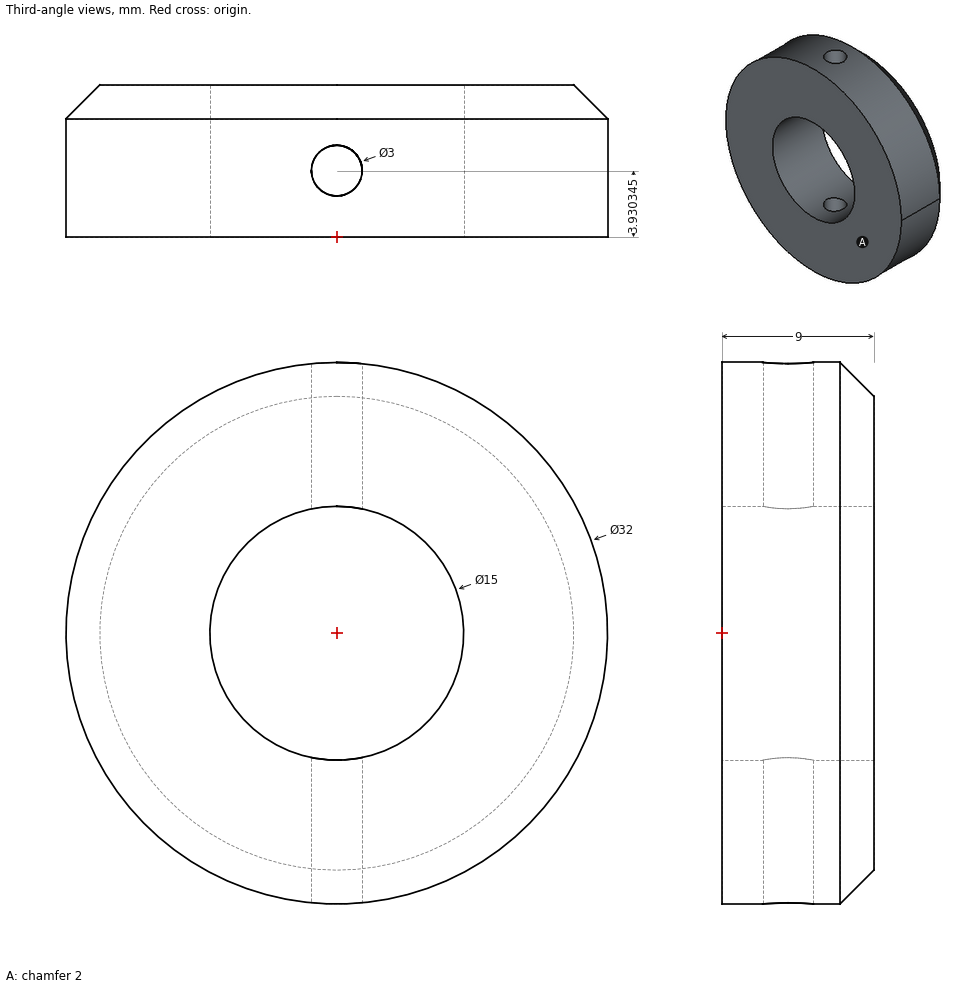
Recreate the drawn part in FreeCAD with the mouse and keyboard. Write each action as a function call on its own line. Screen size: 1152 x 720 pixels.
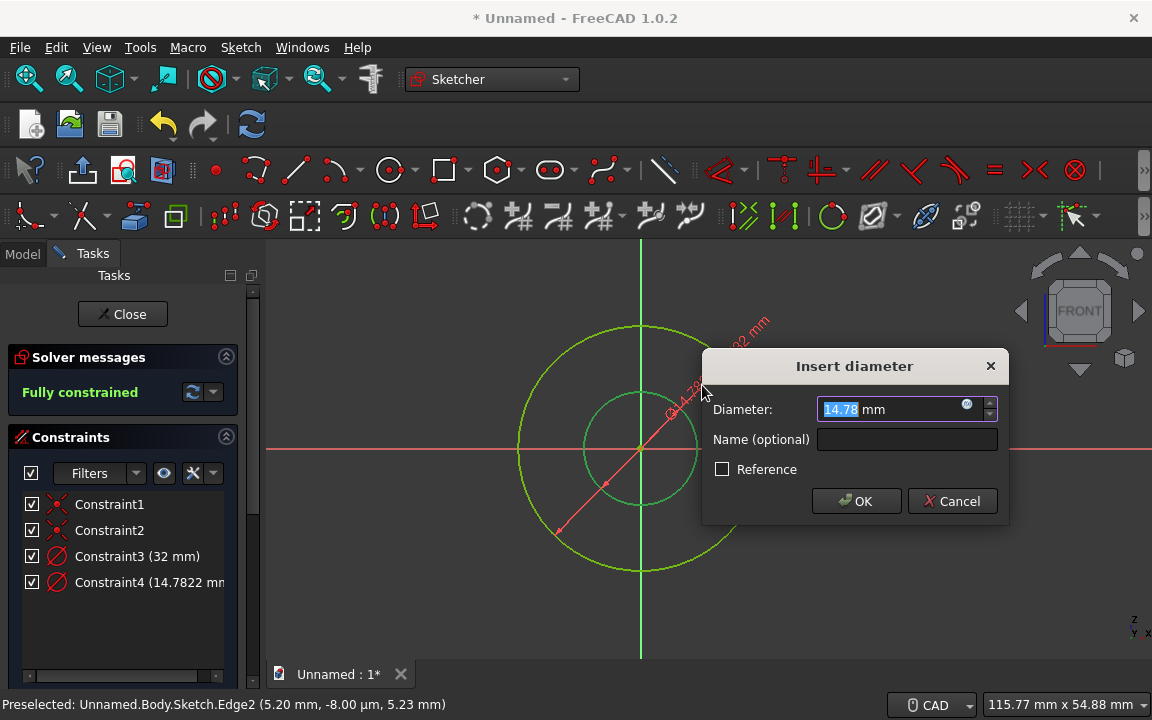
text(15)
key(Return)
key(Escape)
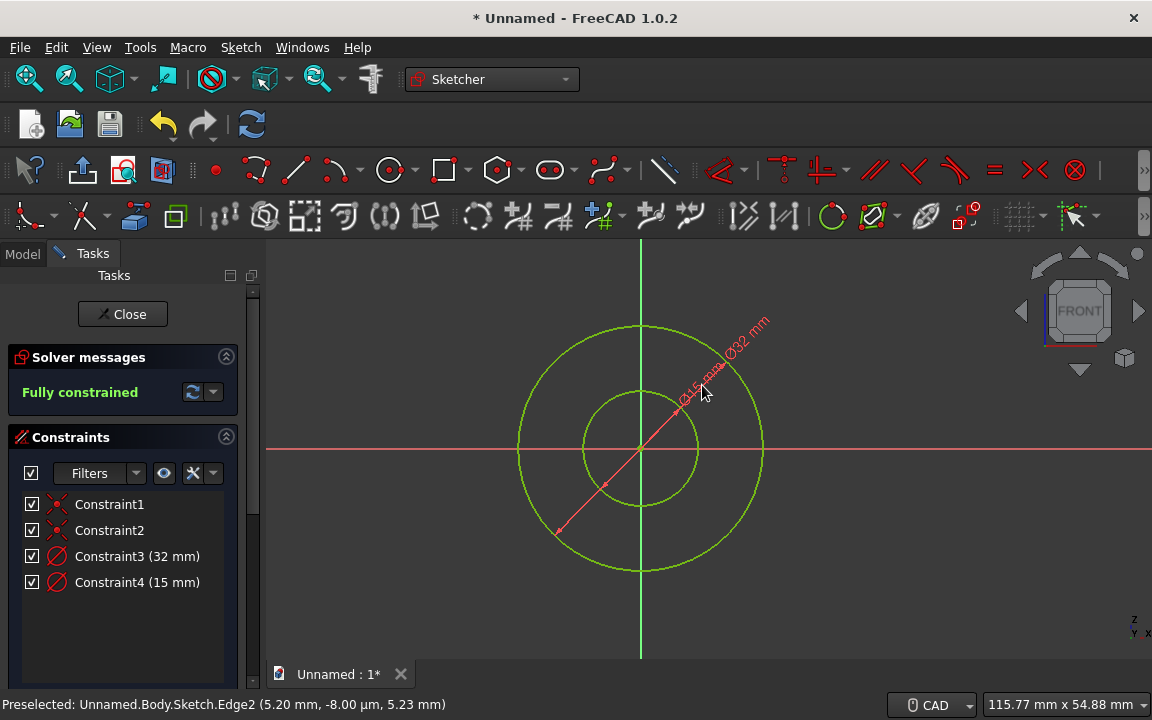
click(123, 314)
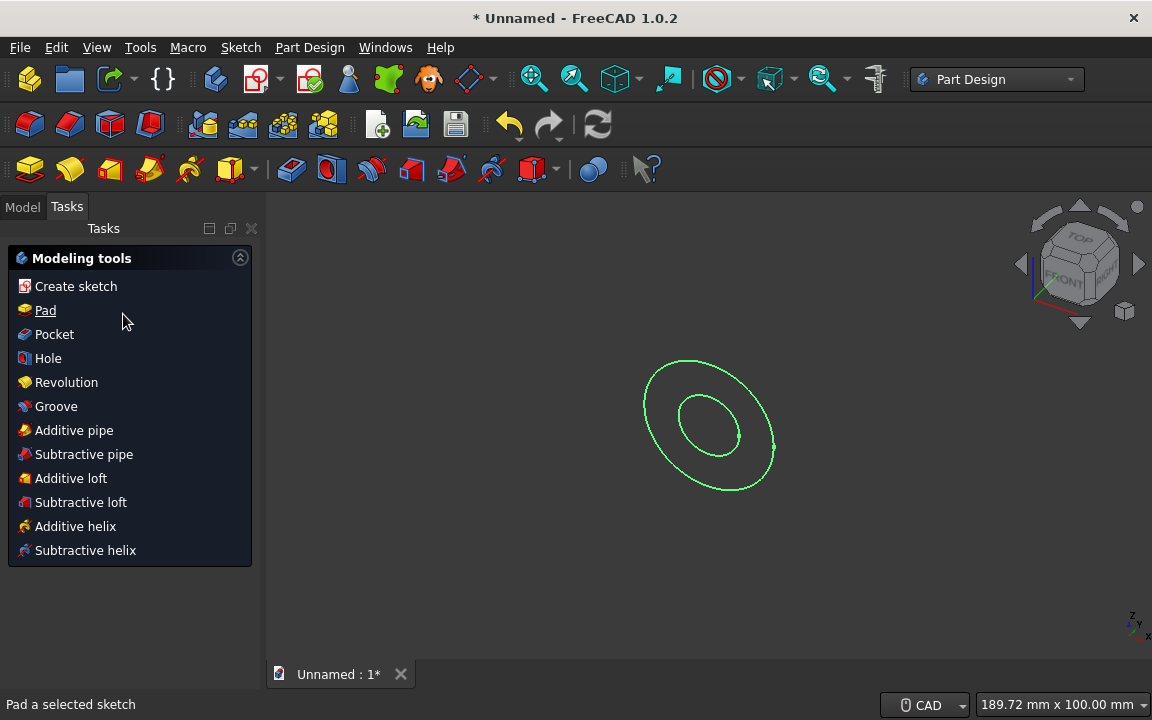
click(30, 170)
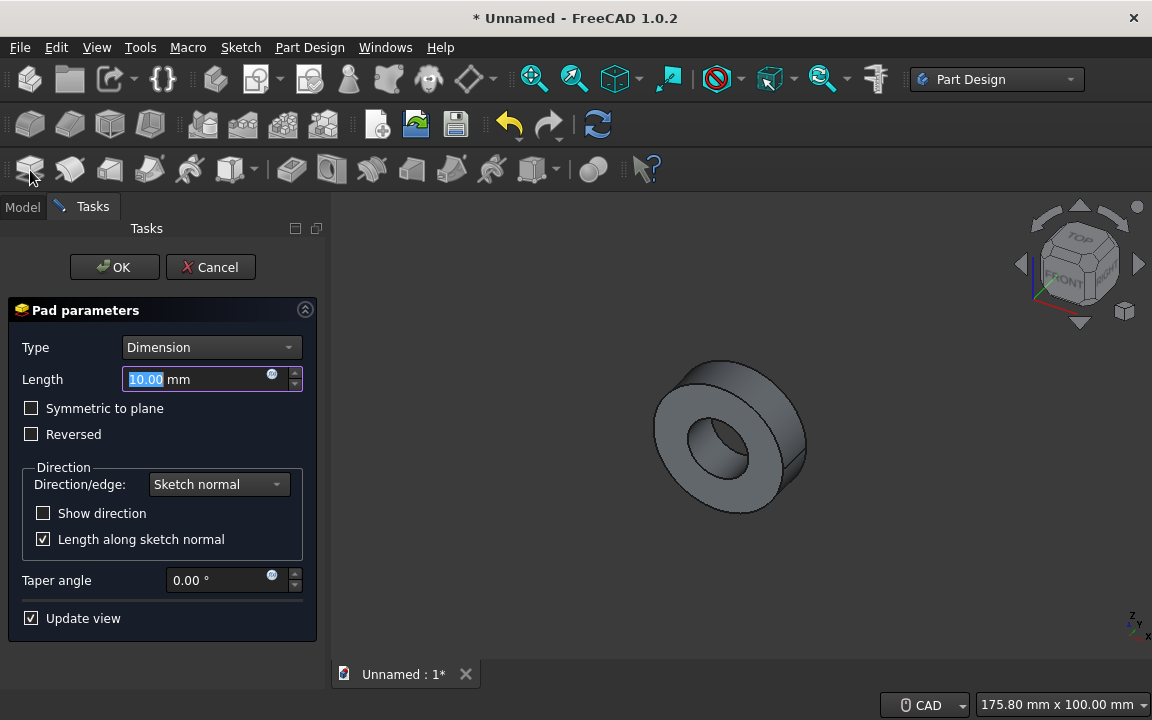
text(9)
key(Tab)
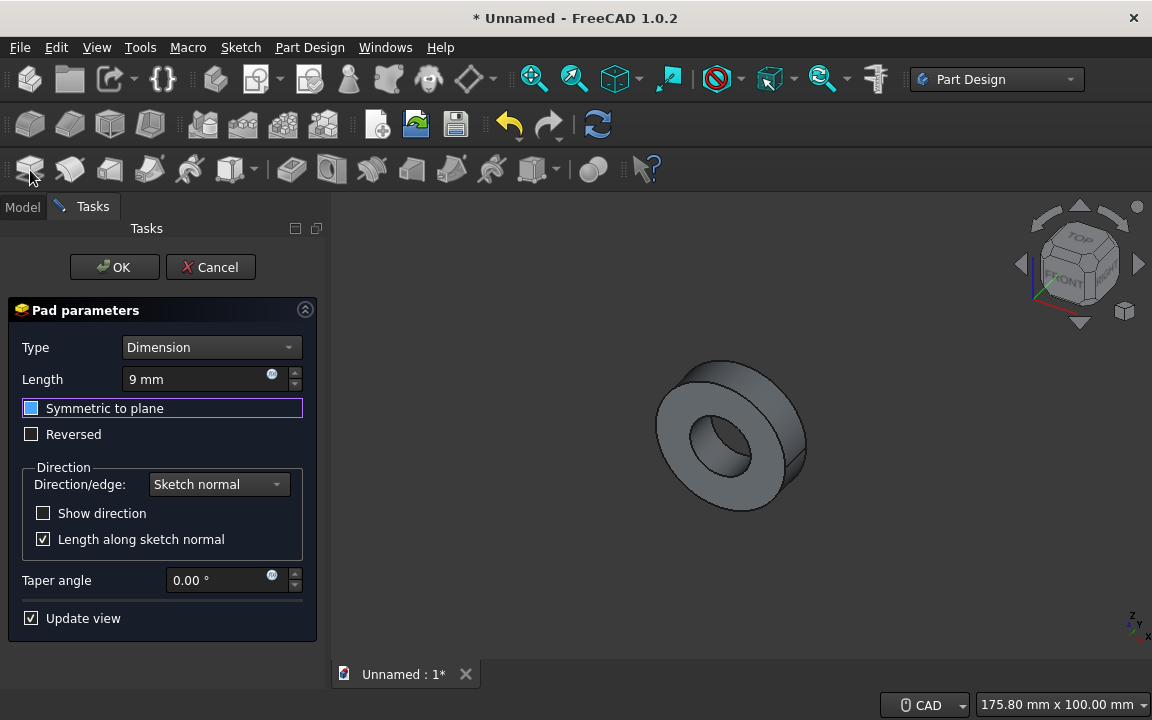
click(30, 434)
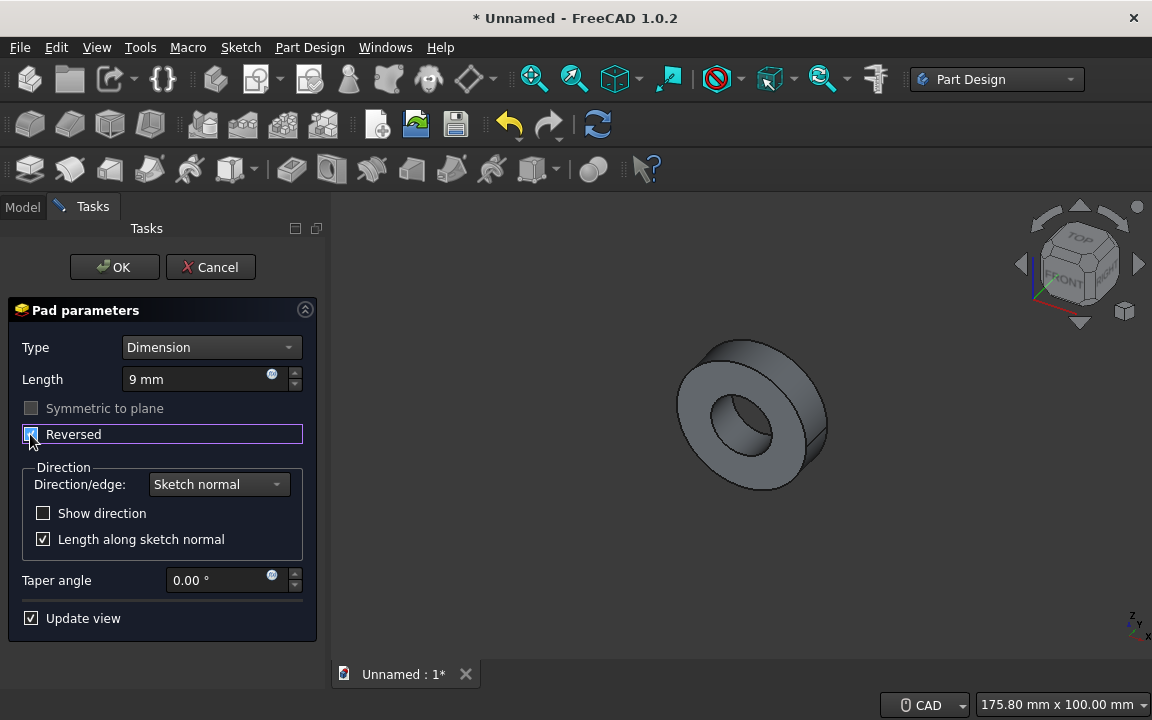
click(115, 267)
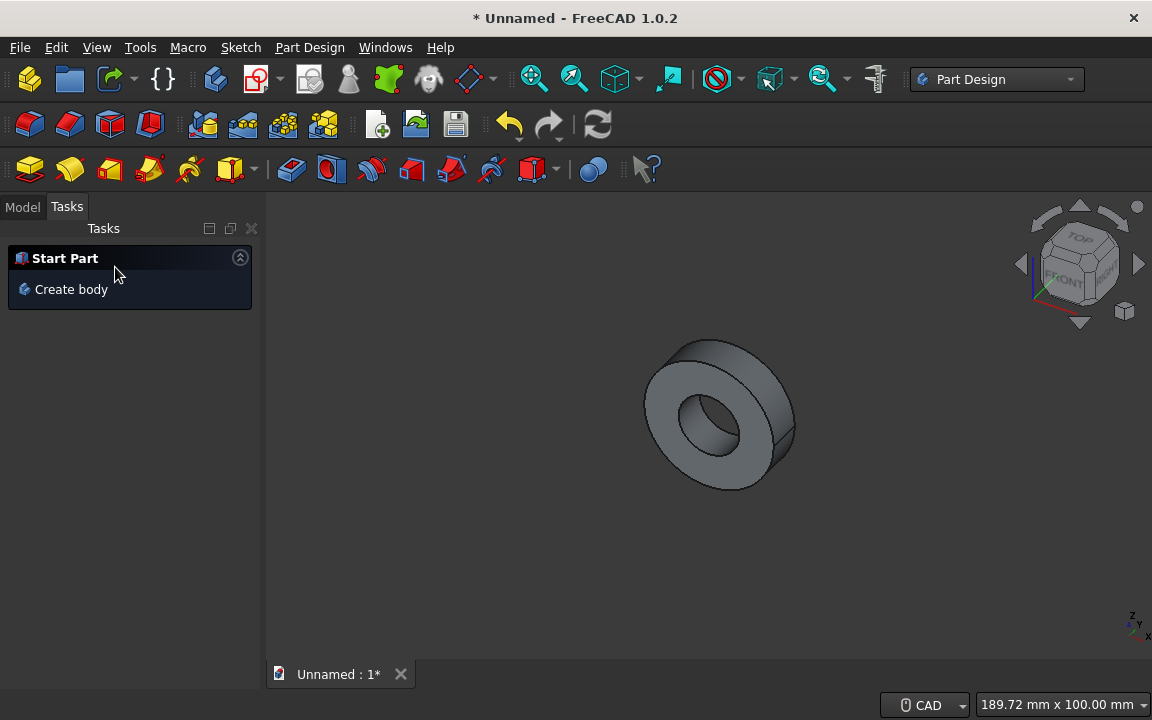
click(536, 80)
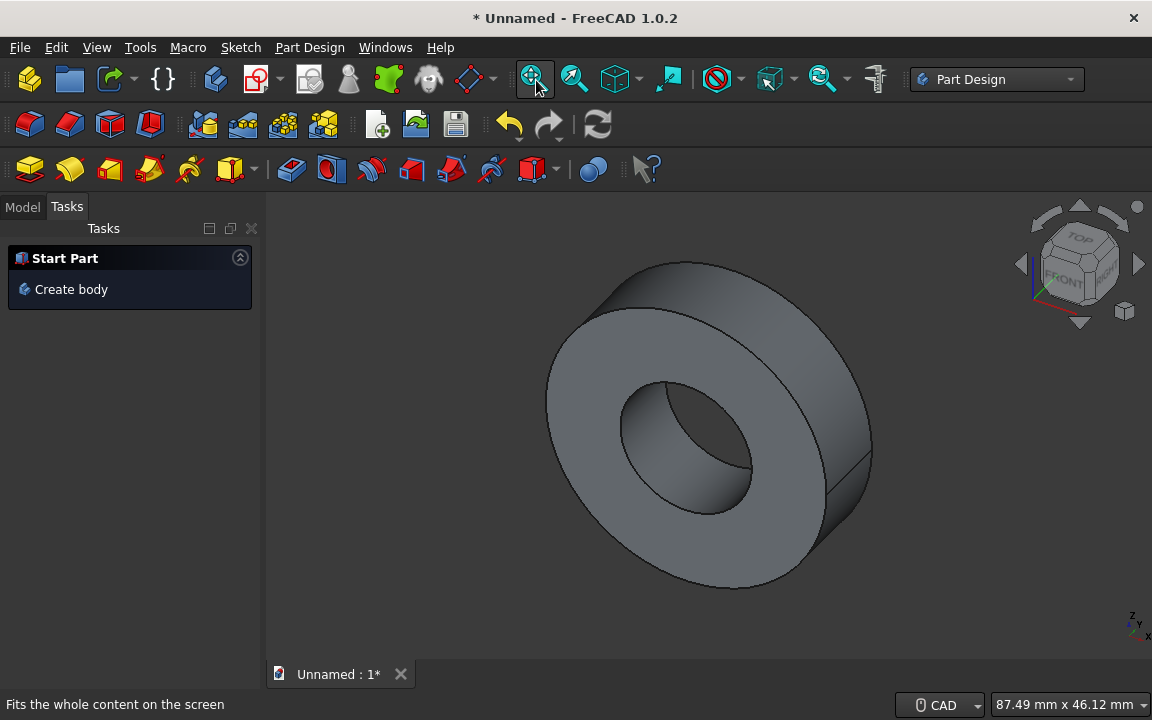
key(0)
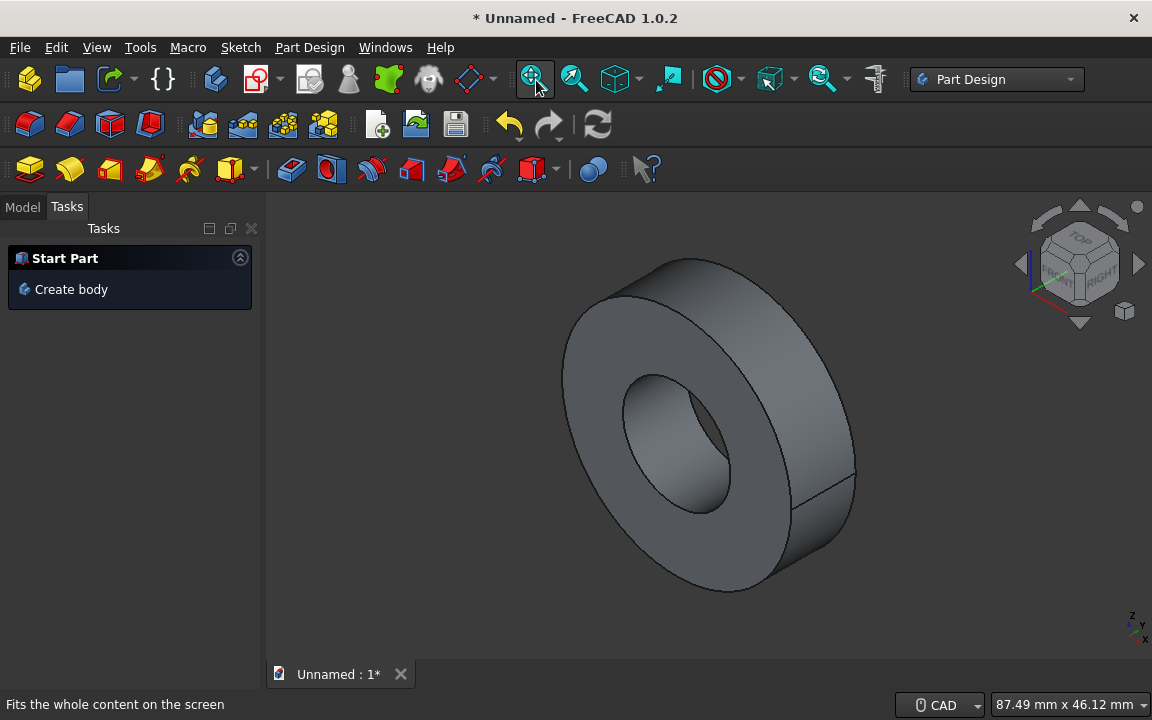
key(2)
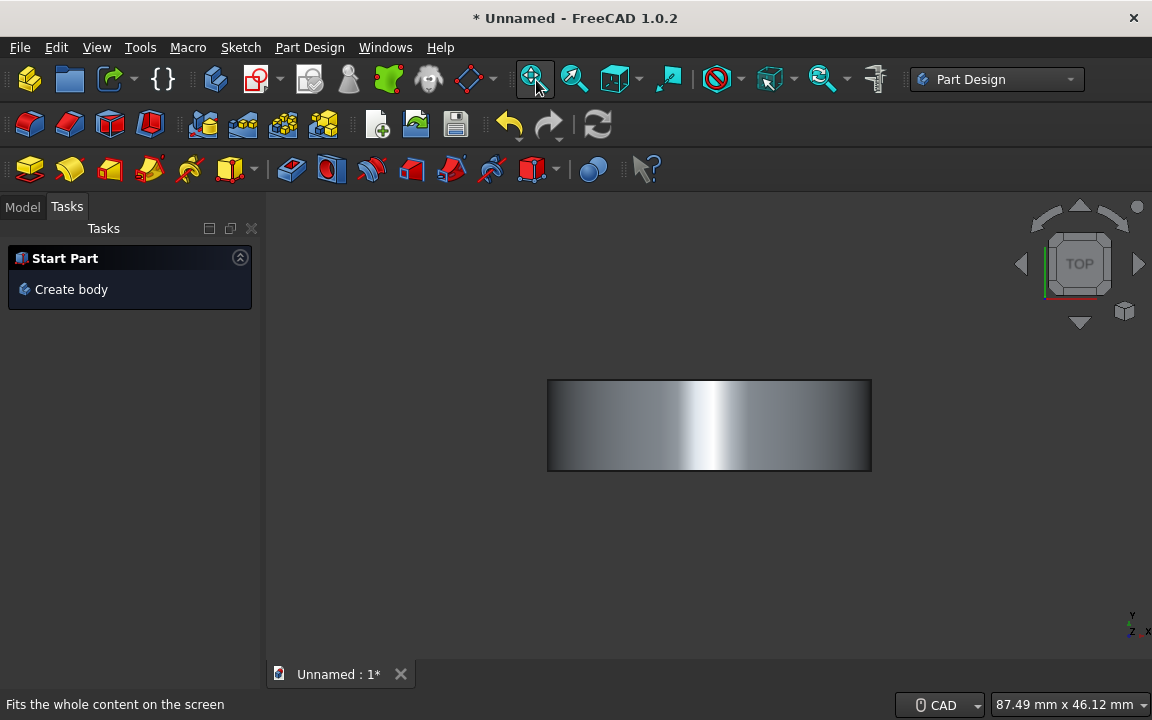
key(v)
key(f)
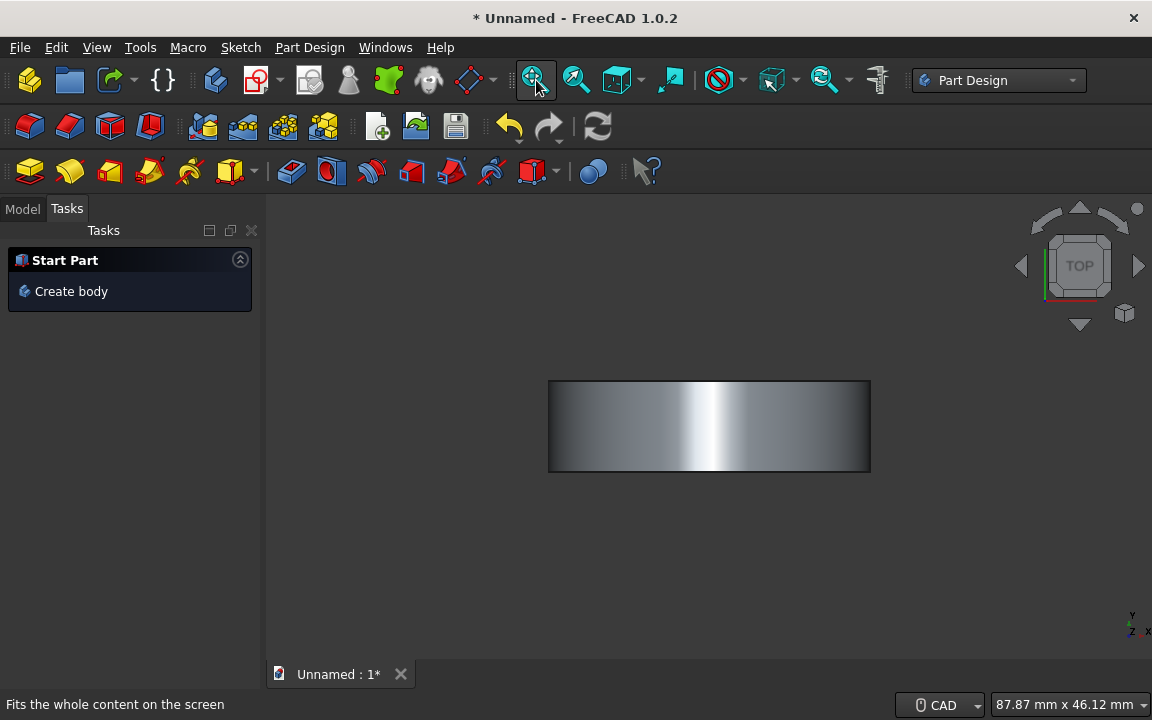
click(578, 380)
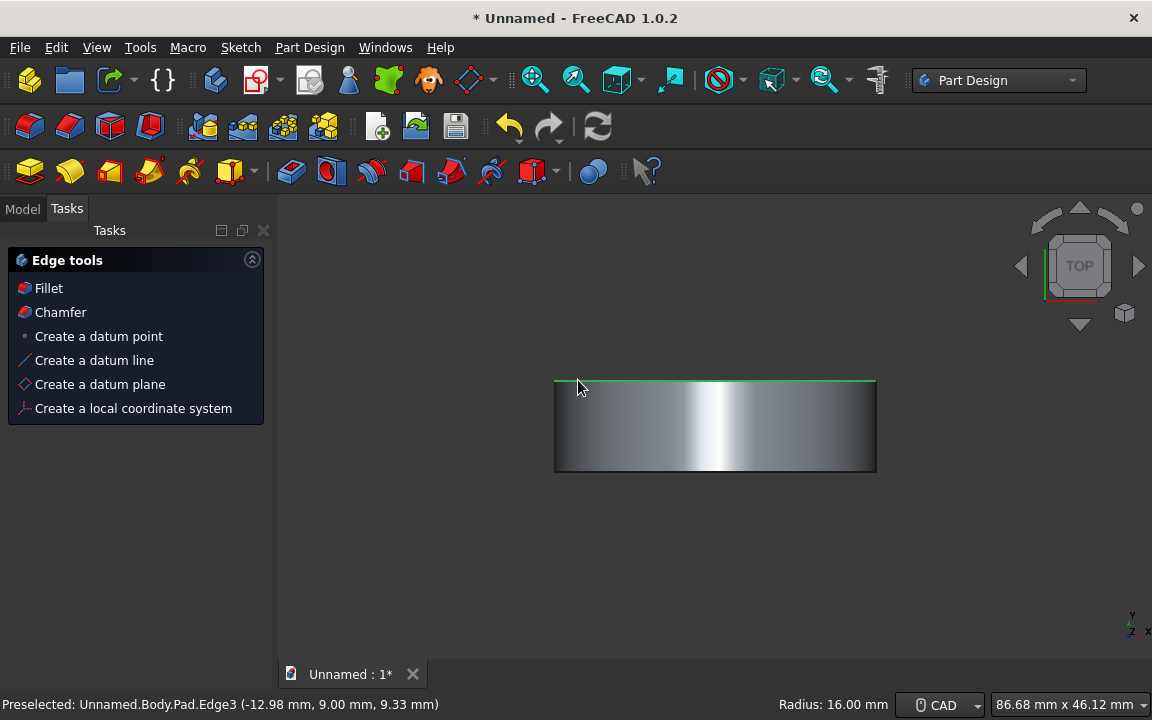
click(70, 126)